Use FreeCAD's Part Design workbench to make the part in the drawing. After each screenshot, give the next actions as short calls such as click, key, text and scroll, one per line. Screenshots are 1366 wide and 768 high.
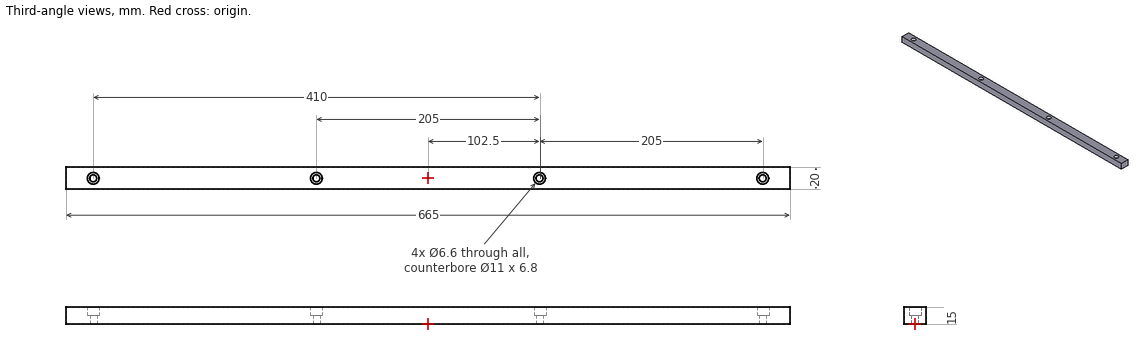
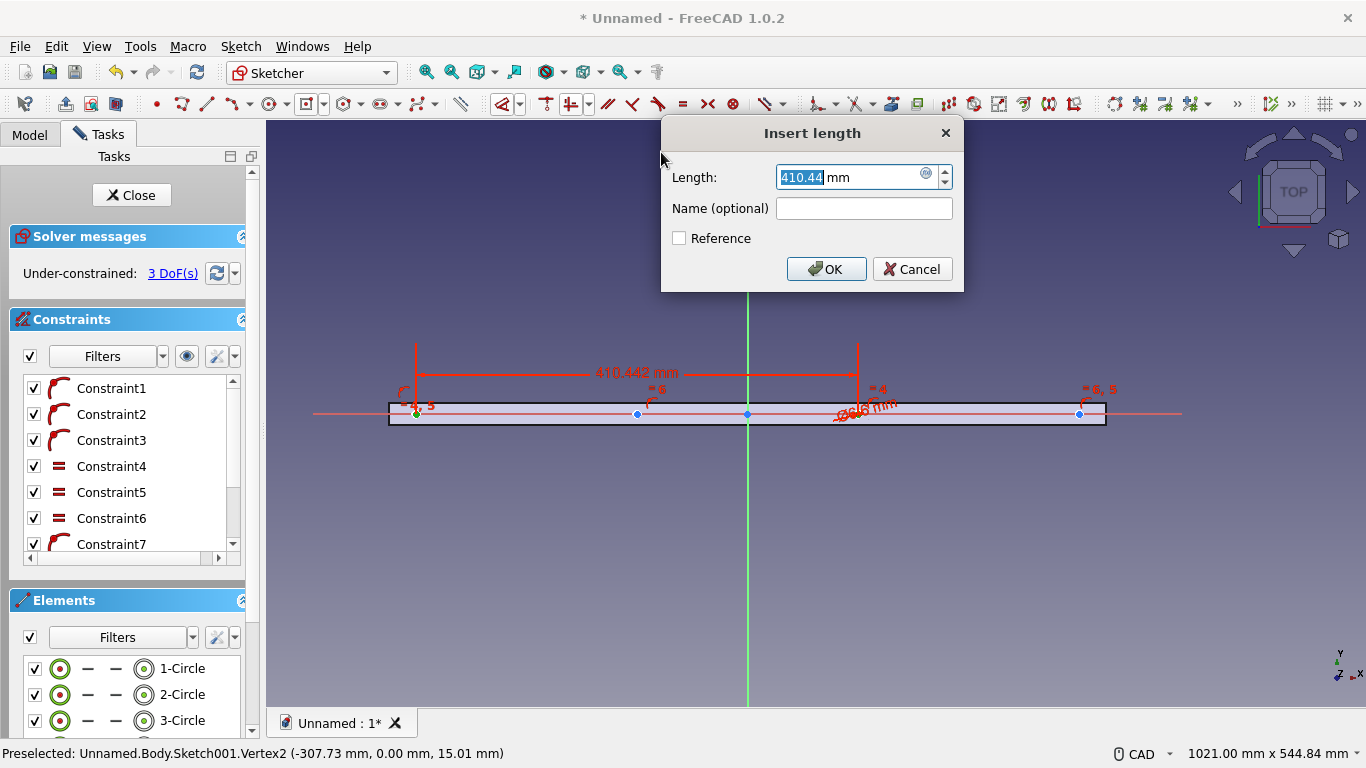
text(410)
key(Return)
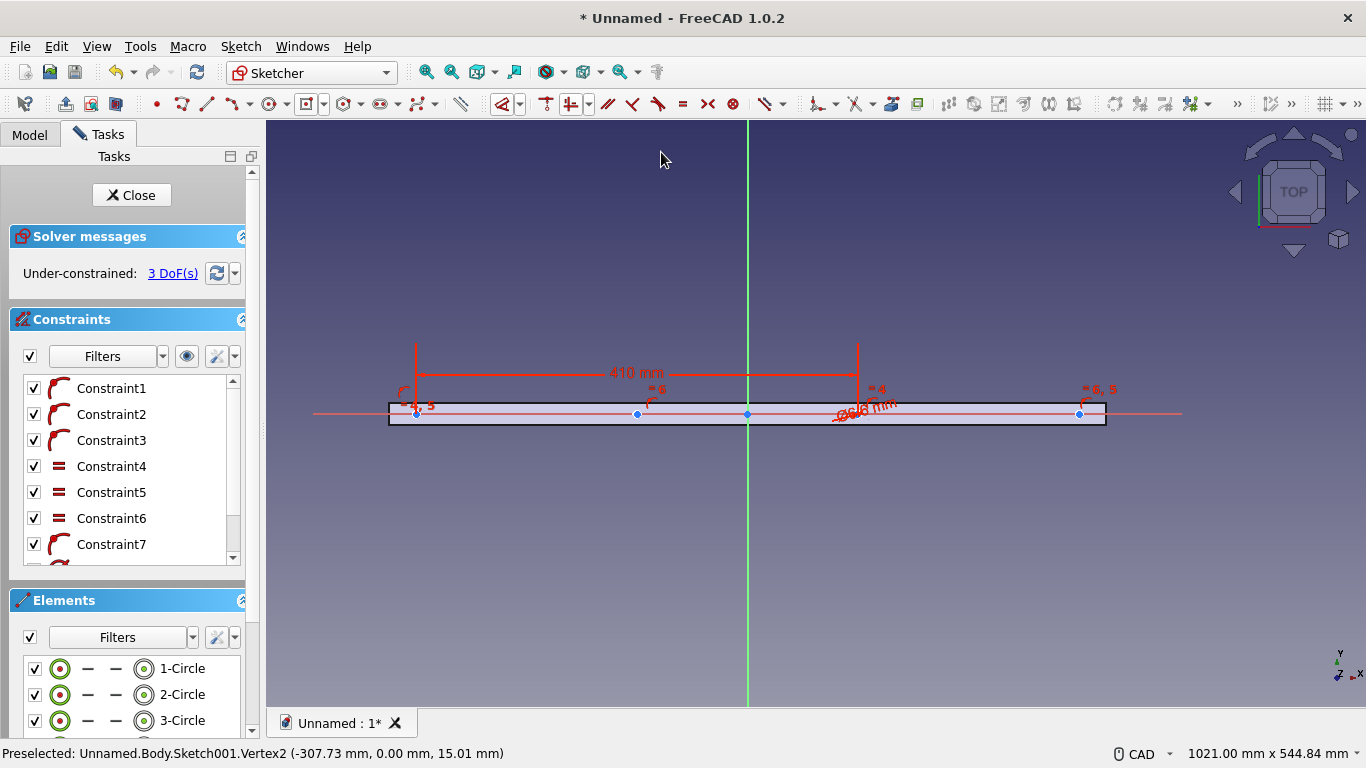
click(858, 414)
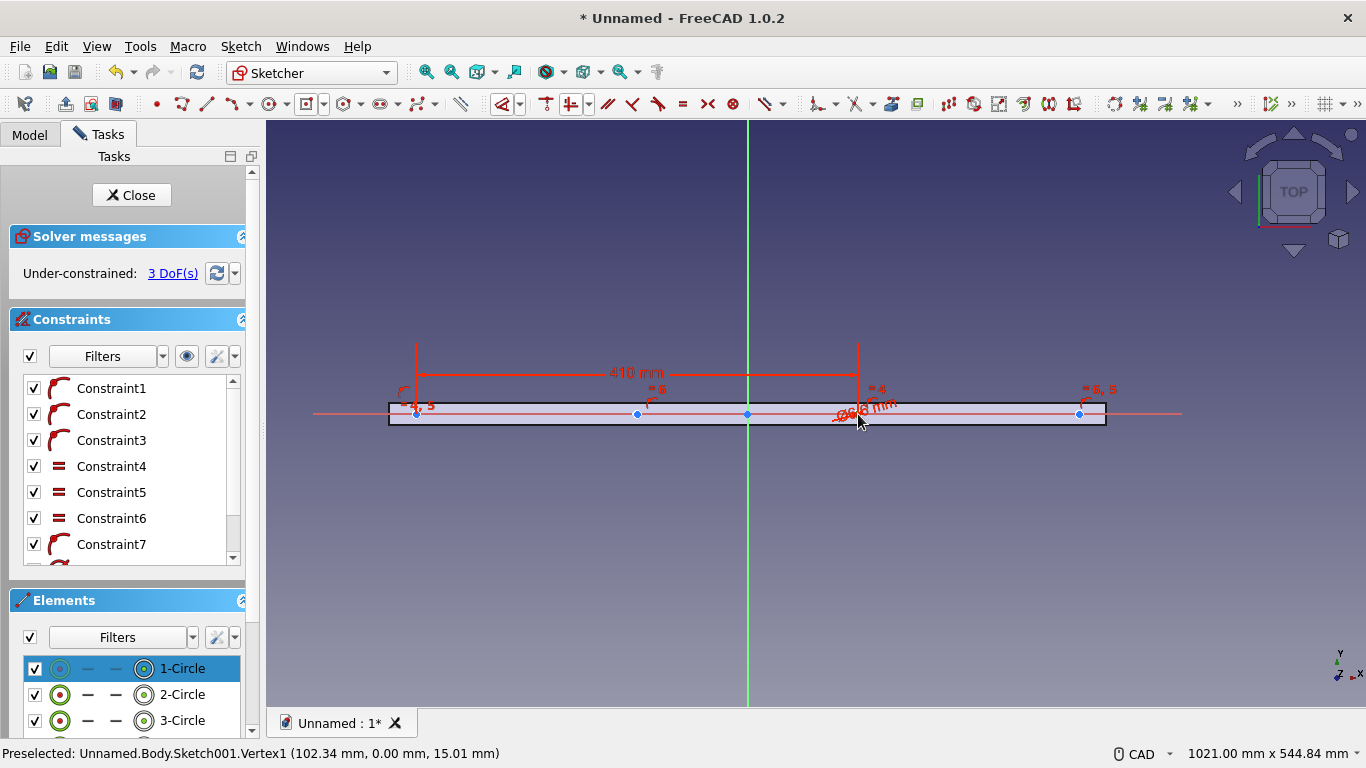
click(1079, 414)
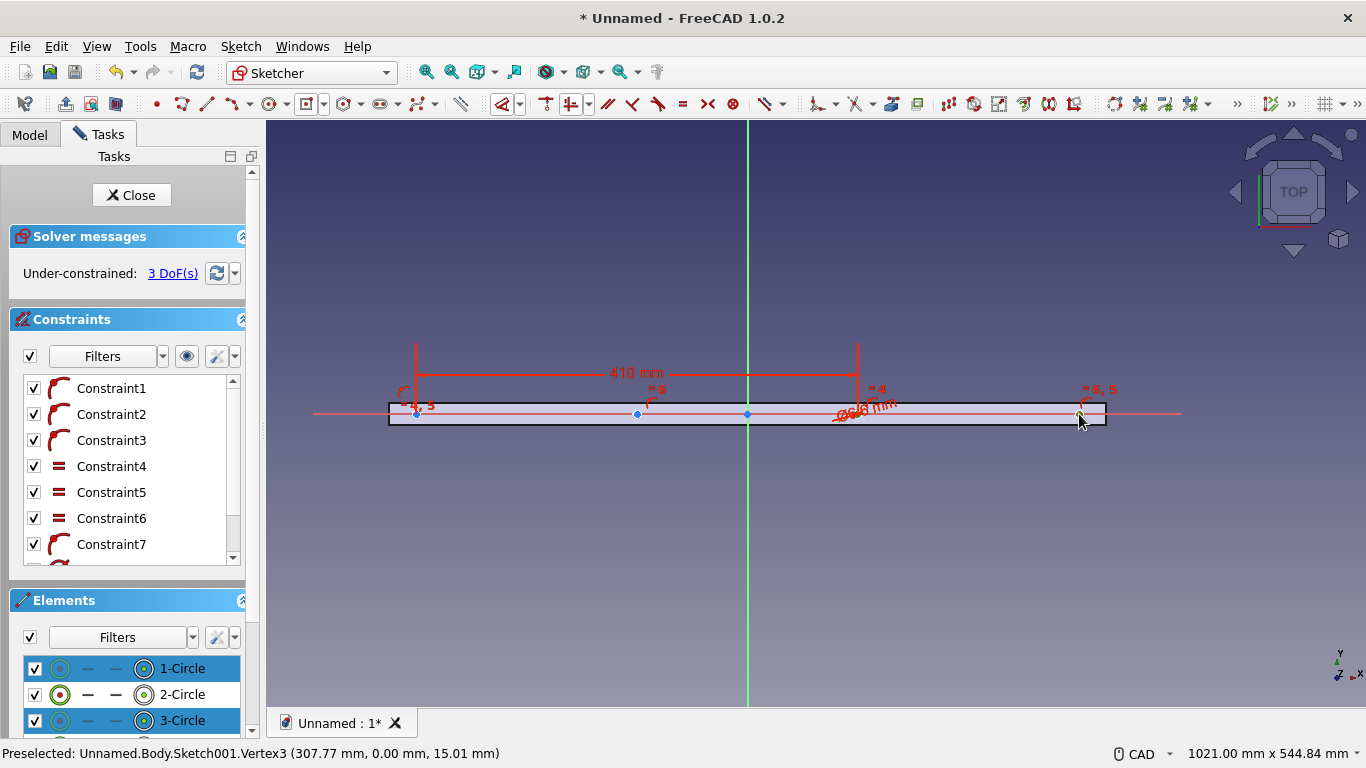
key(l)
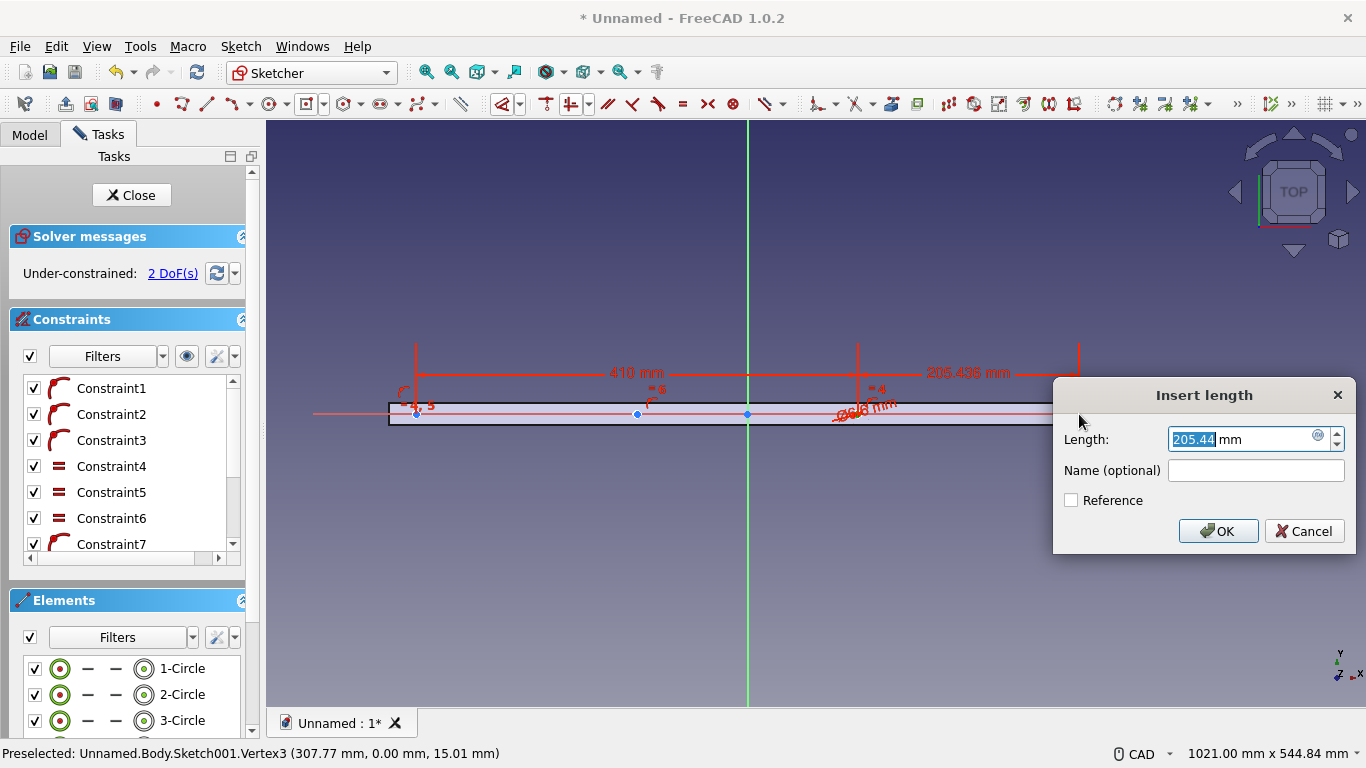
text(205)
key(Return)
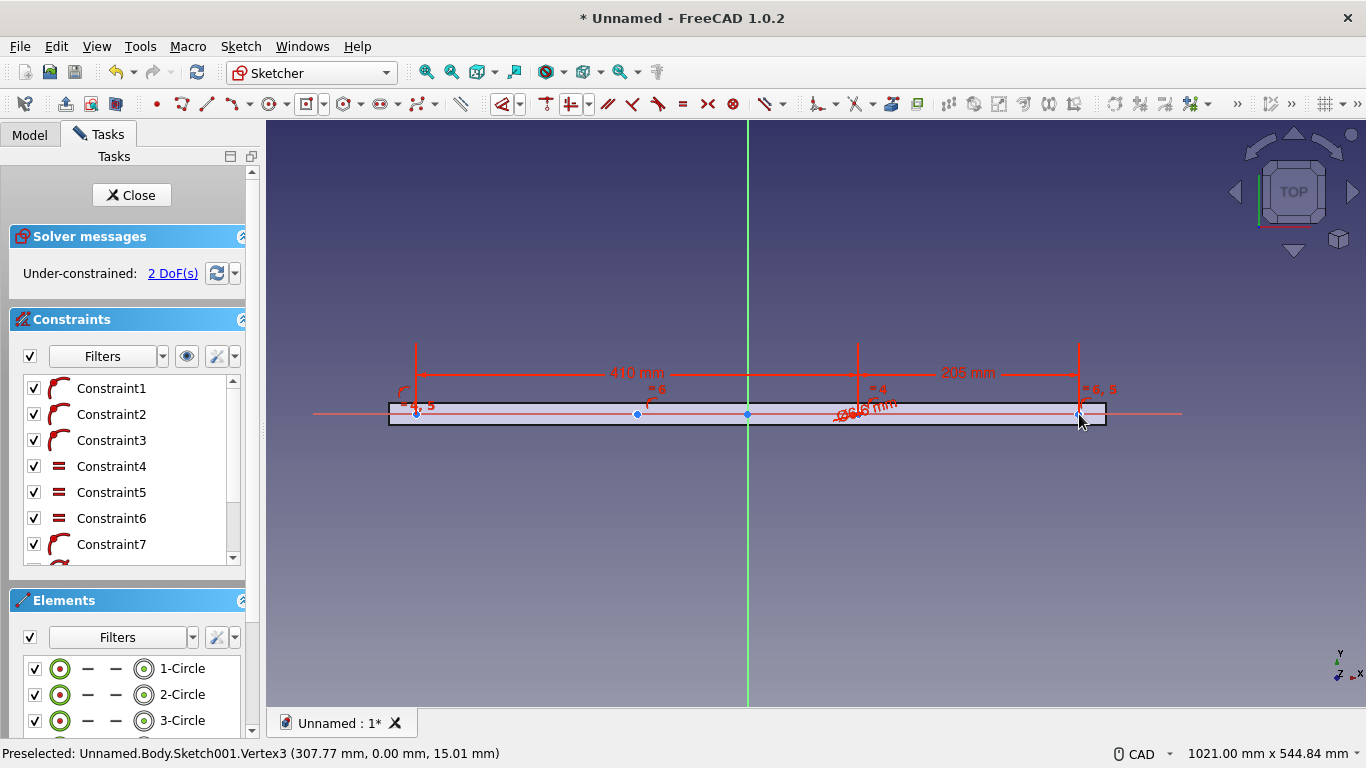
click(858, 414)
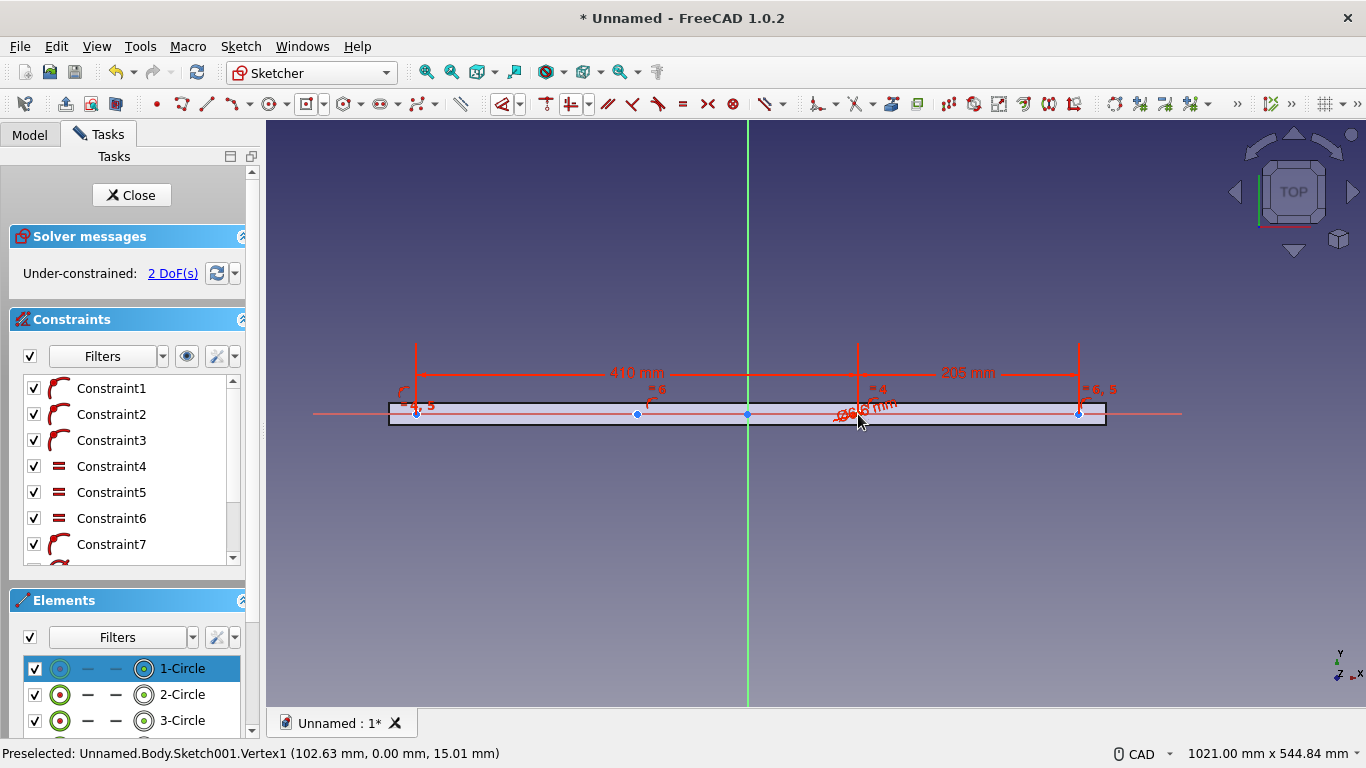
click(637, 414)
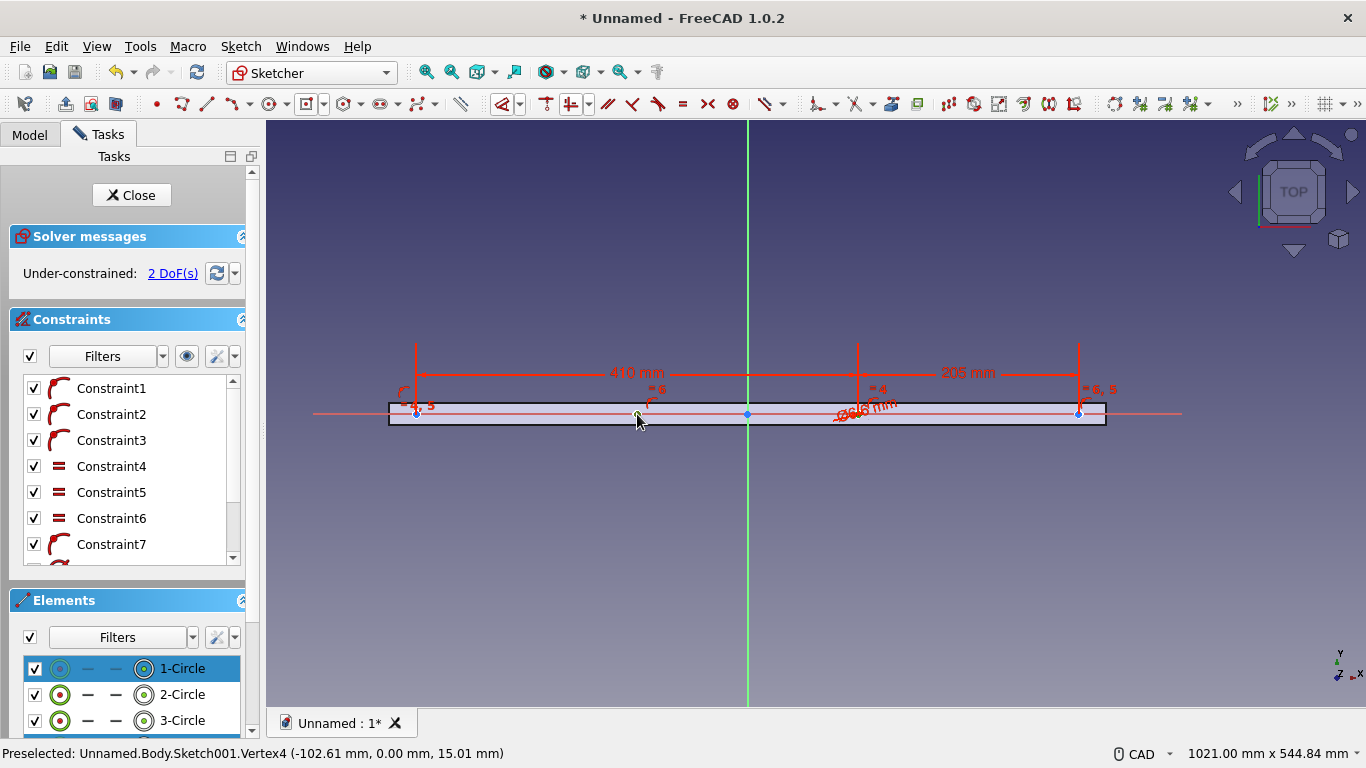
click(520, 104)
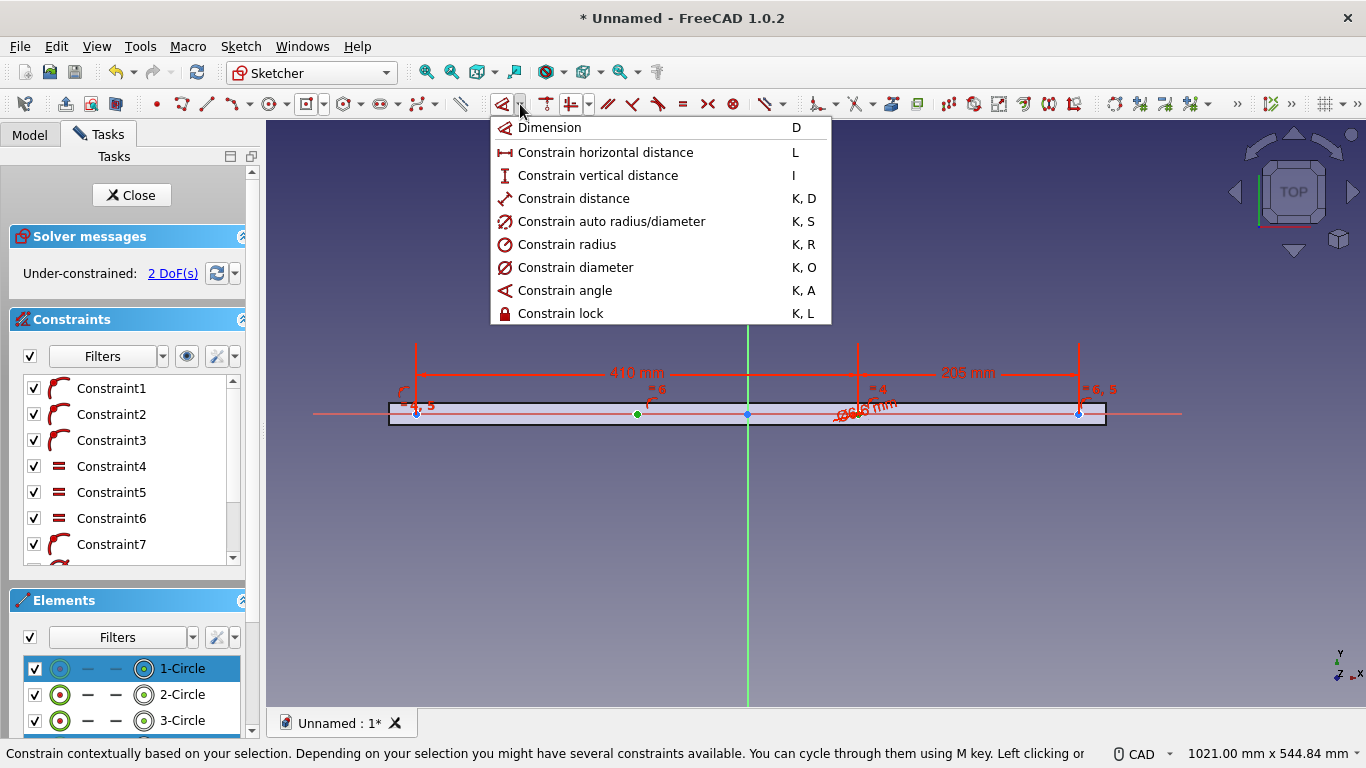
click(661, 152)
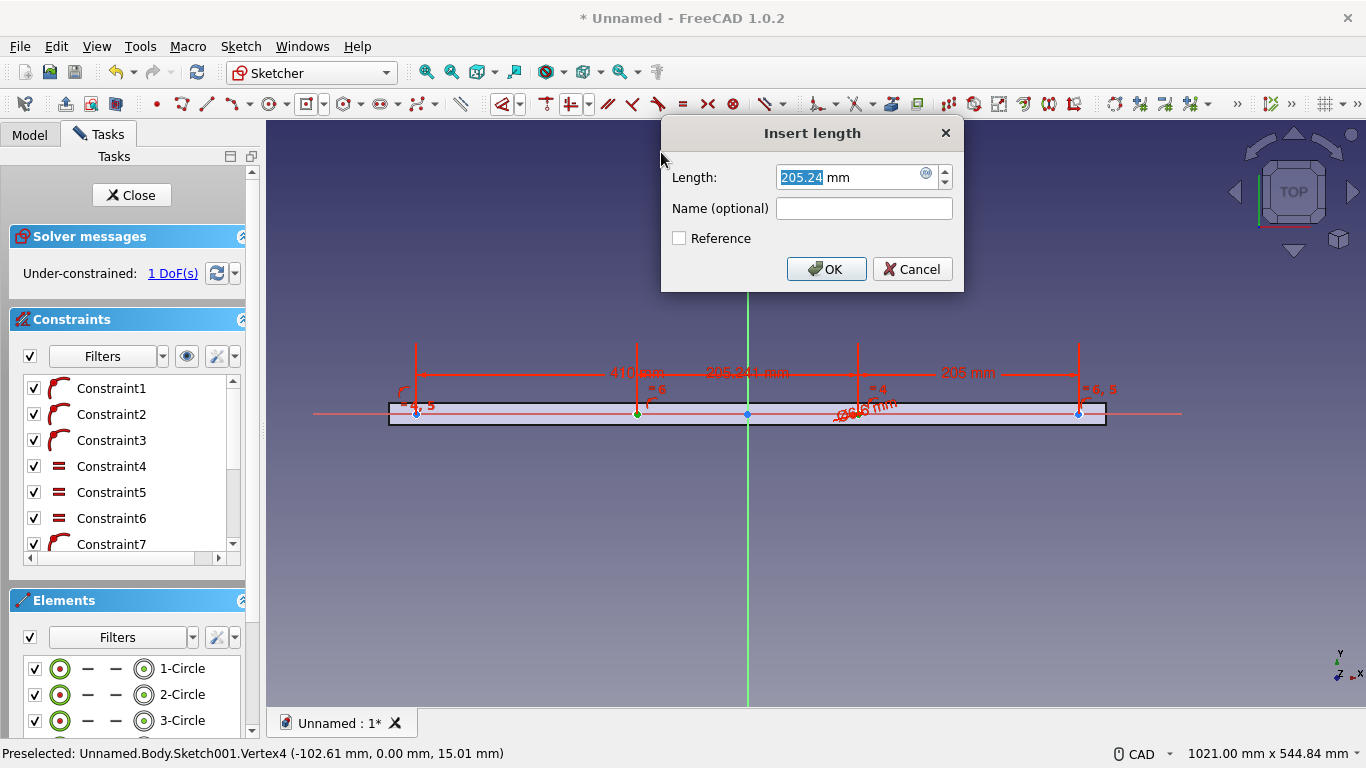
text(205)
key(Return)